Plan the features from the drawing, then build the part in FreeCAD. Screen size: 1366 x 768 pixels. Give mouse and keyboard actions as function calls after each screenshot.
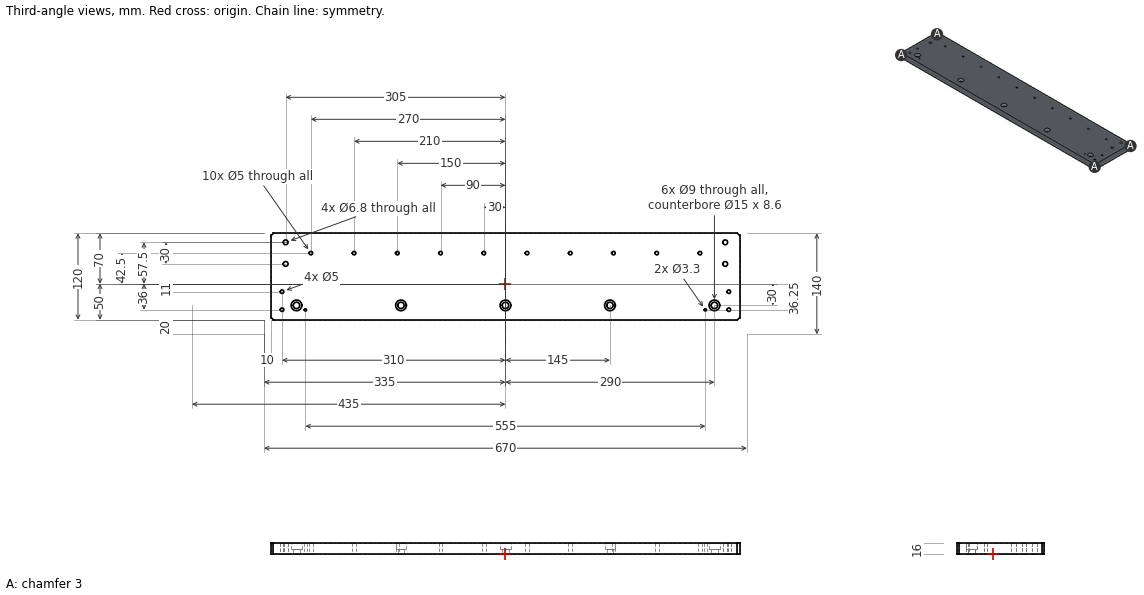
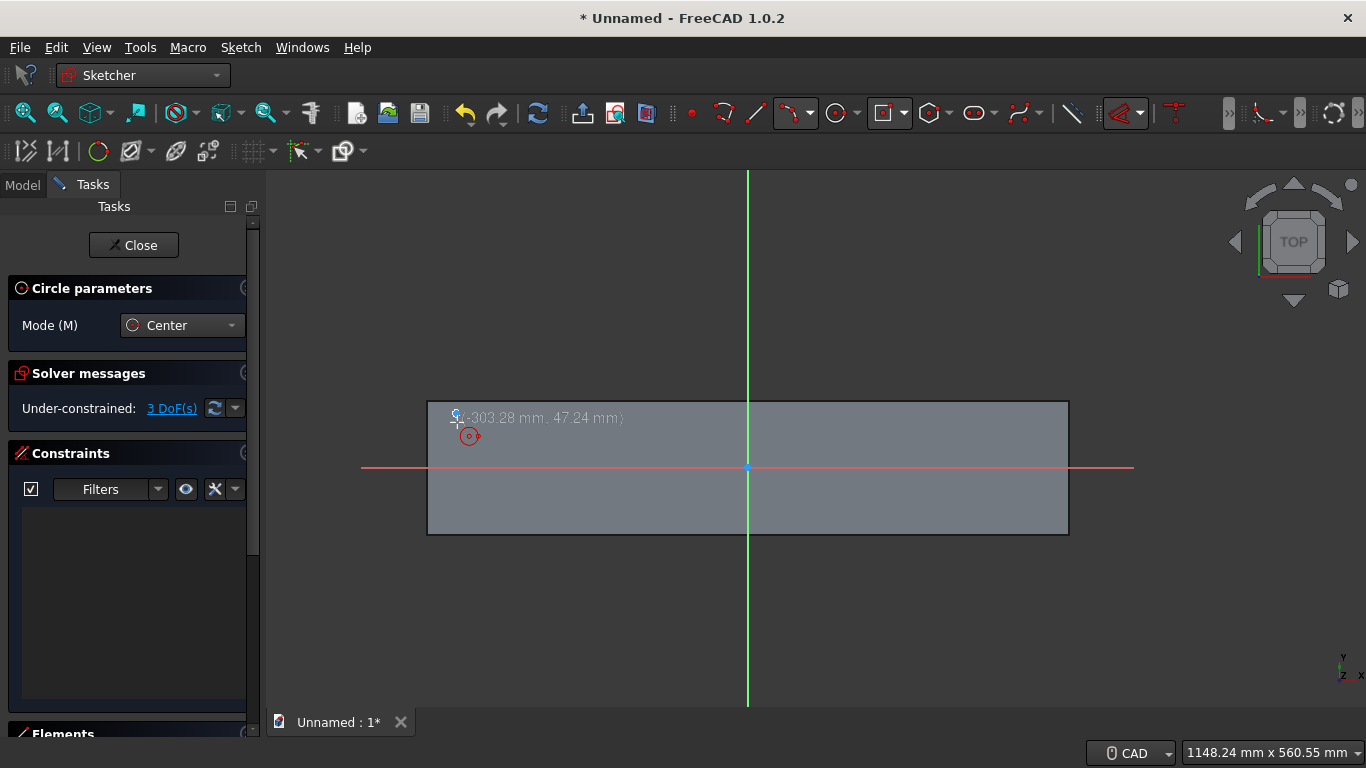
click(456, 441)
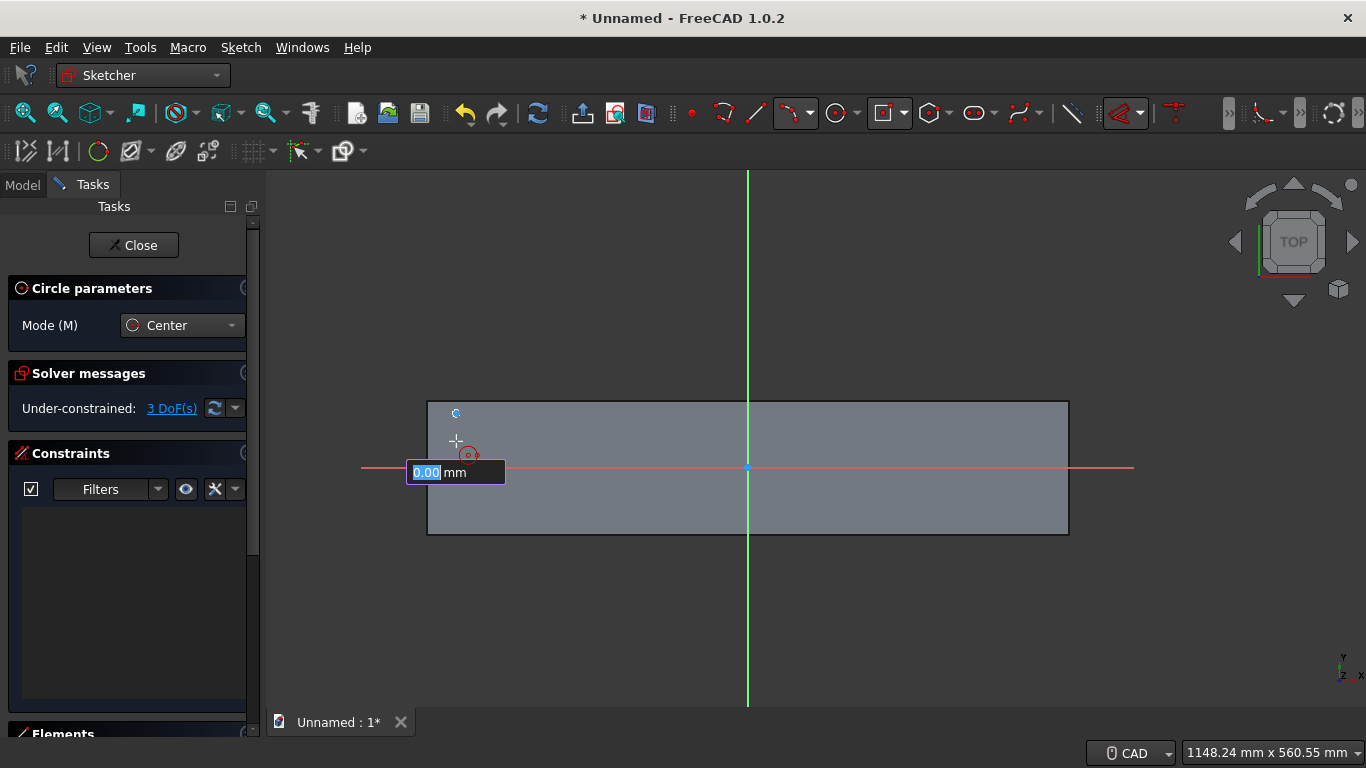
scroll(458, 439, up, 8)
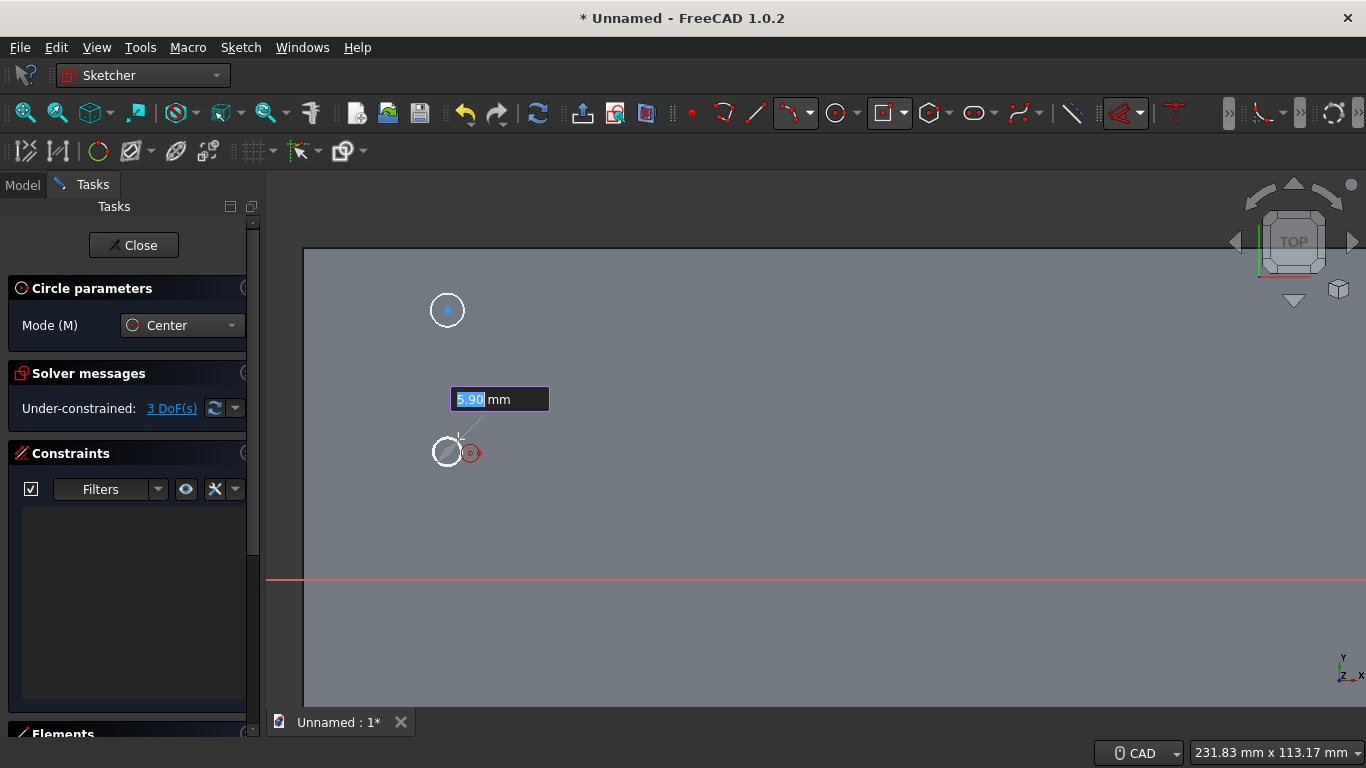
click(456, 438)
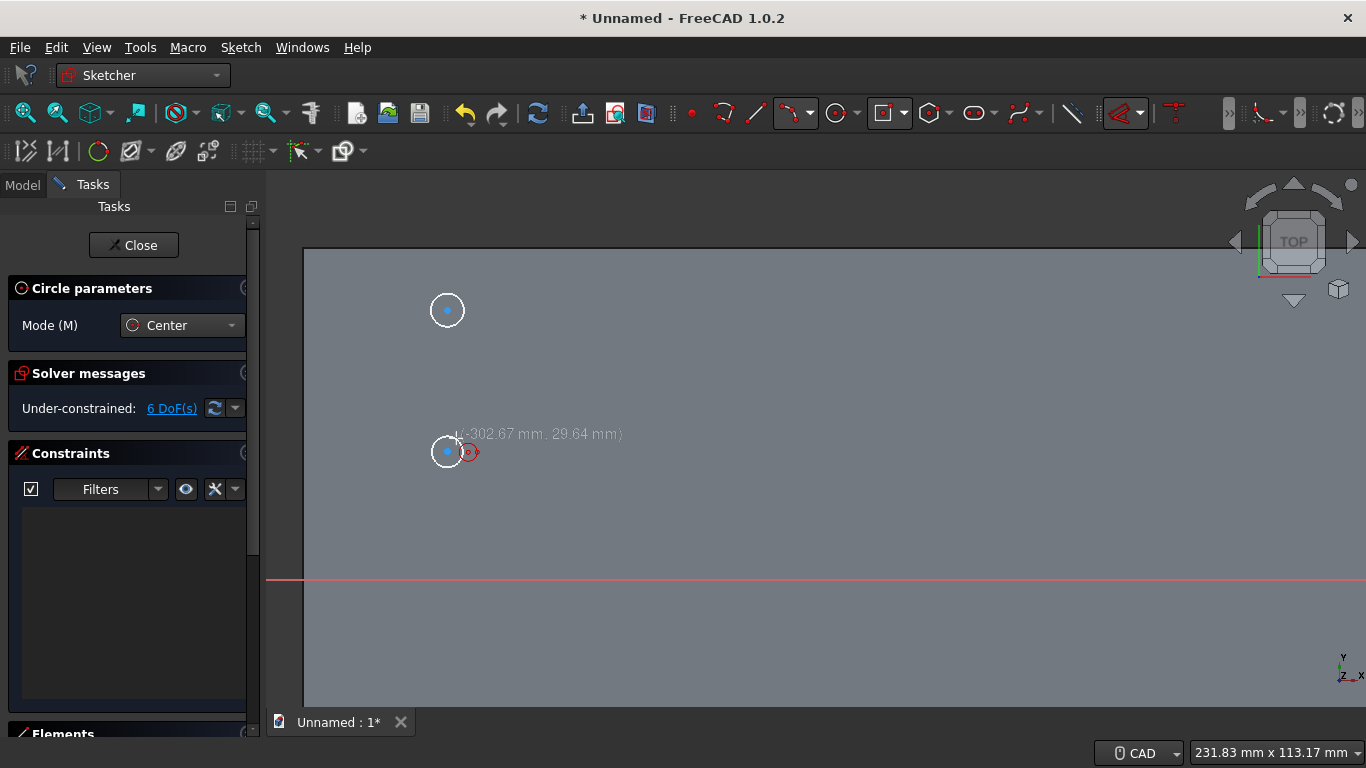
scroll(458, 439, down, 8)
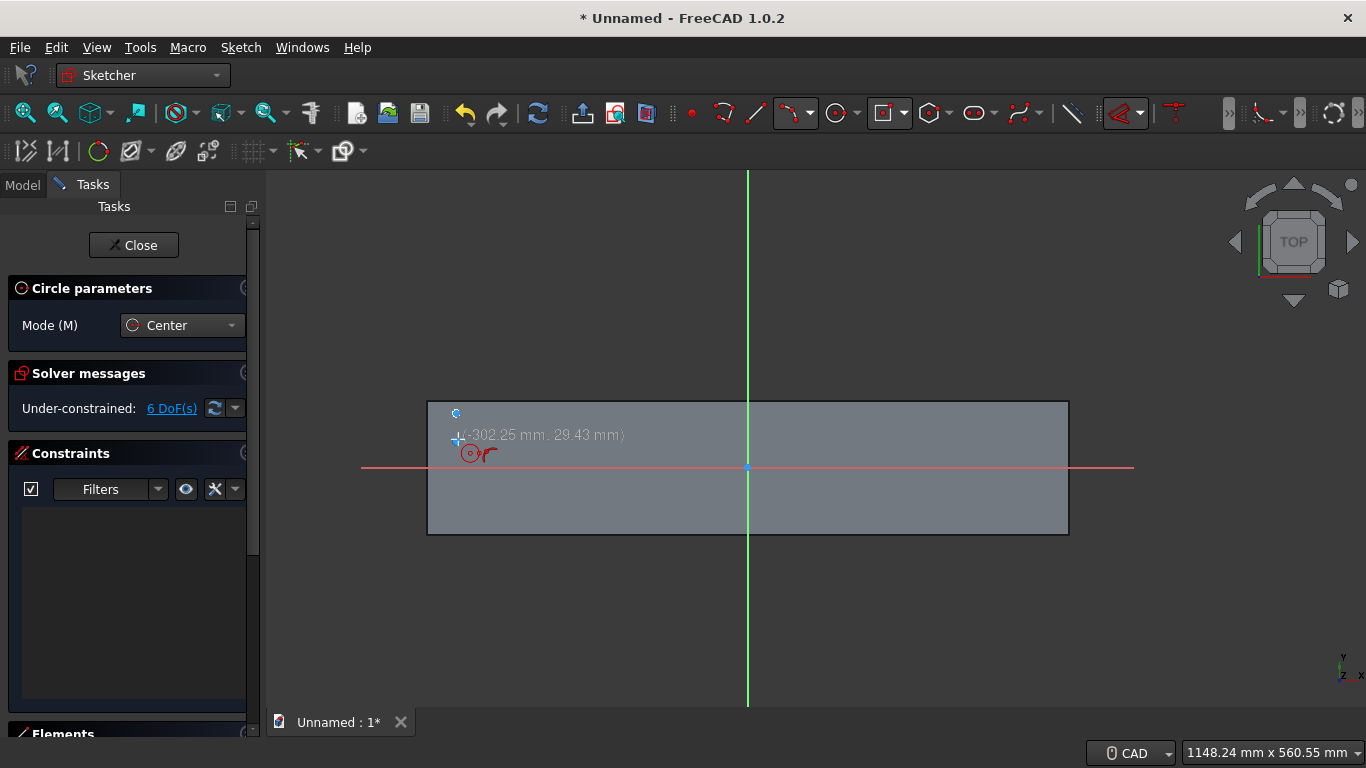
scroll(1040, 441, up, 10)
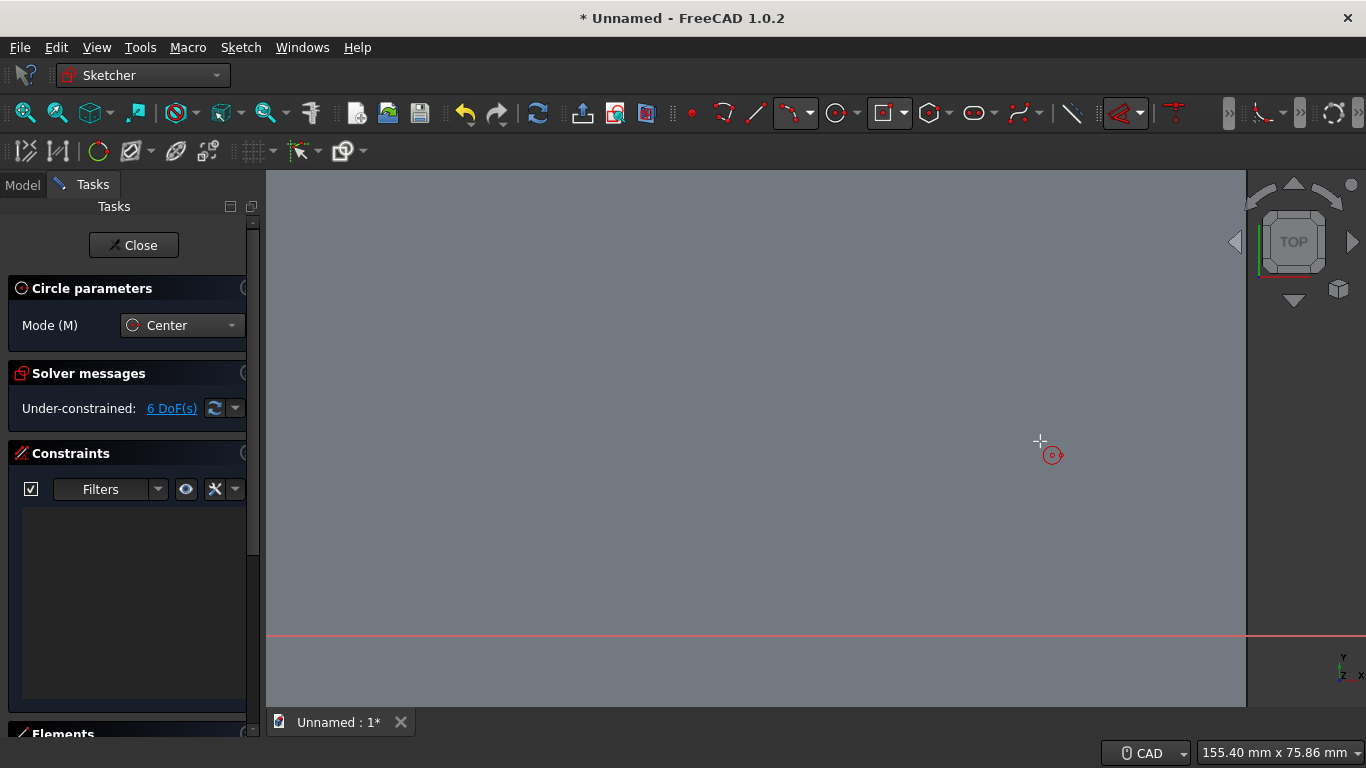
scroll(1040, 441, down, 10)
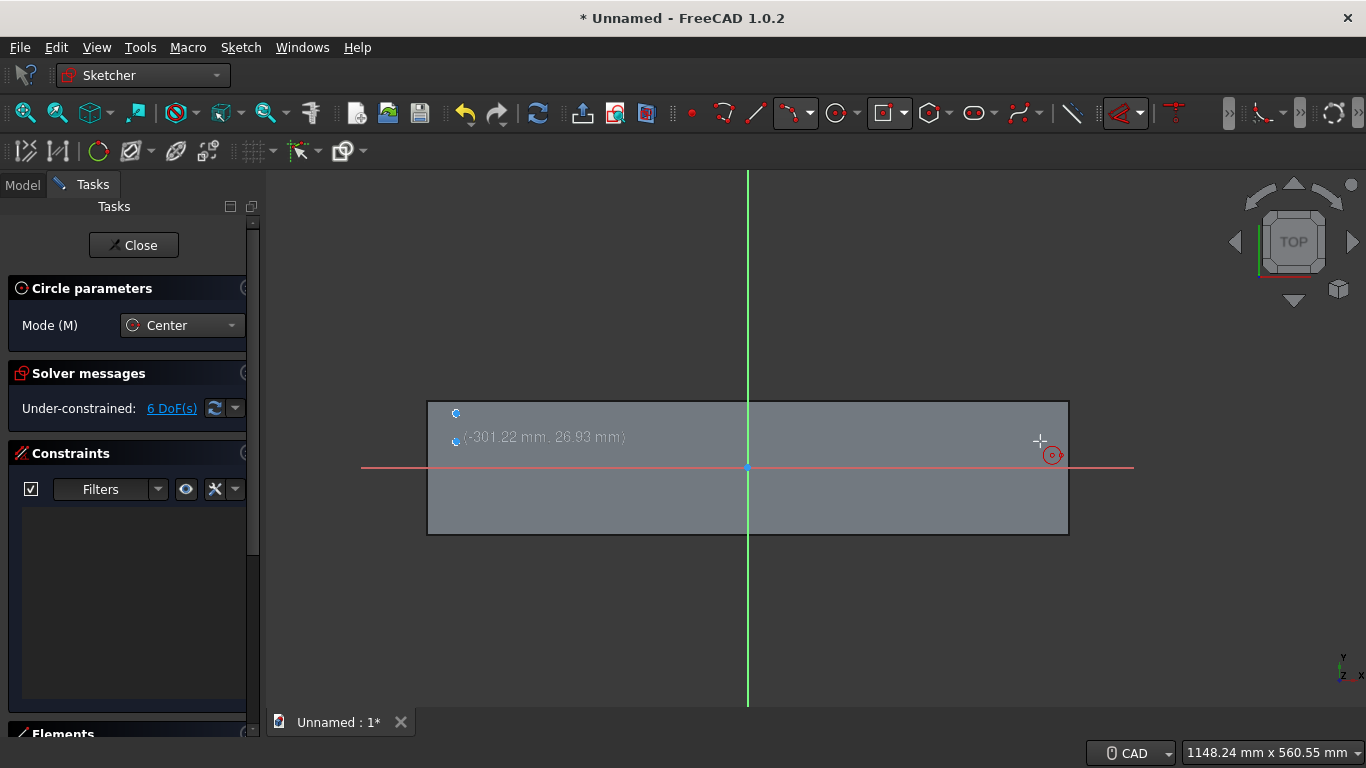
click(1040, 441)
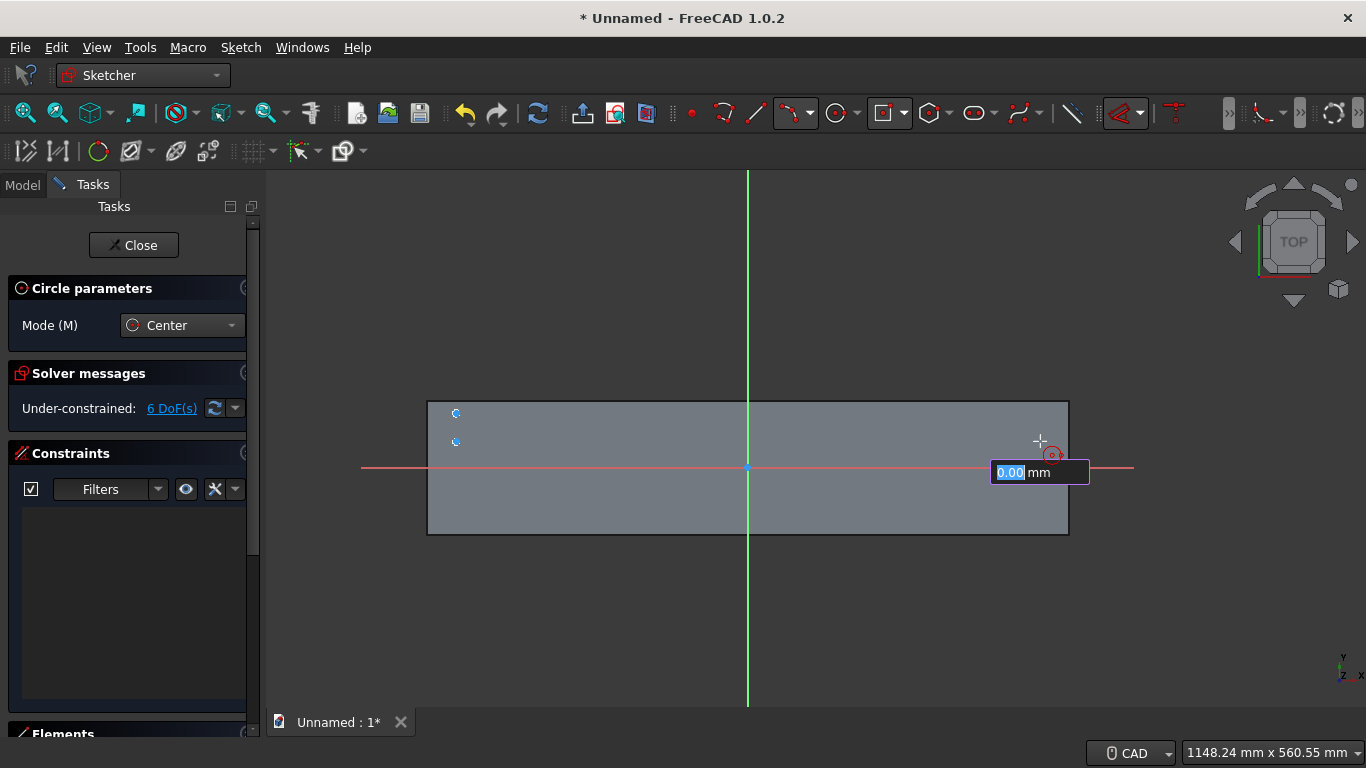
scroll(1042, 439, up, 8)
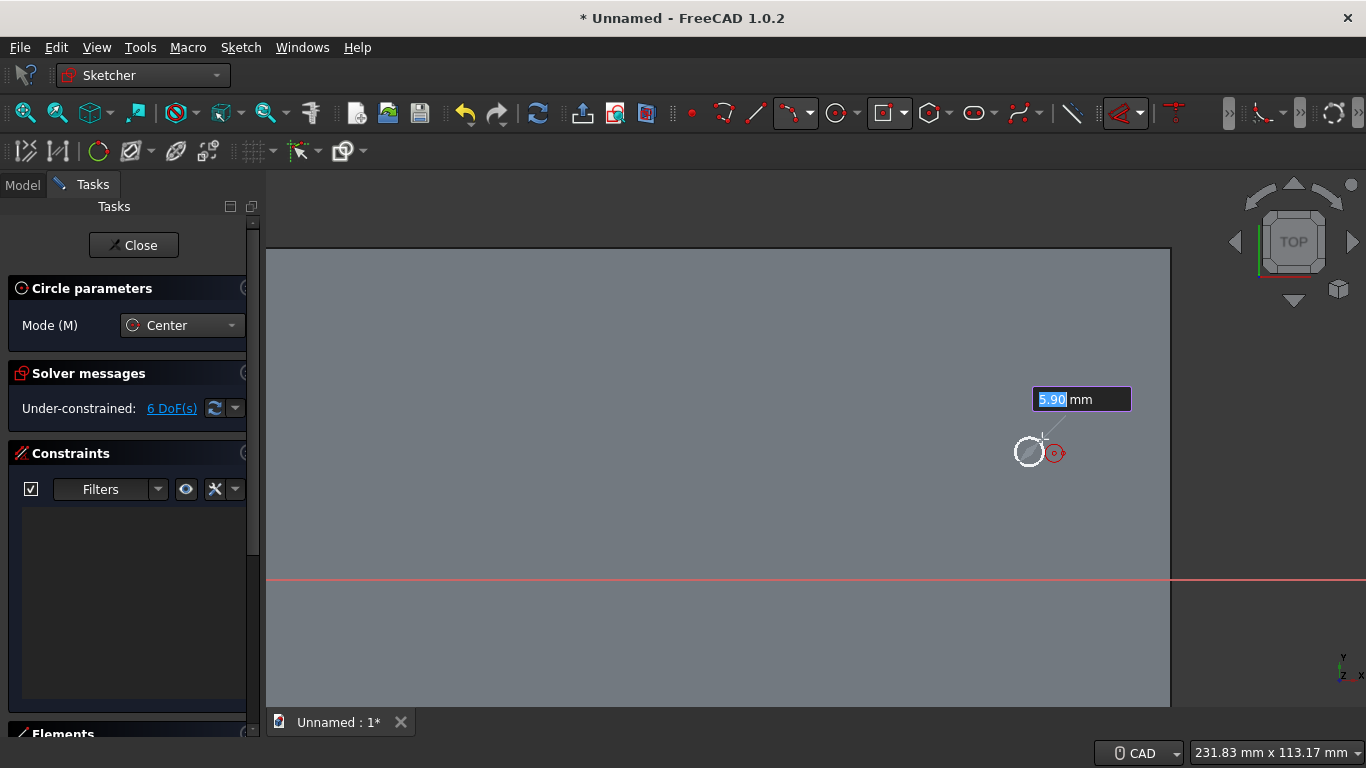
click(1040, 438)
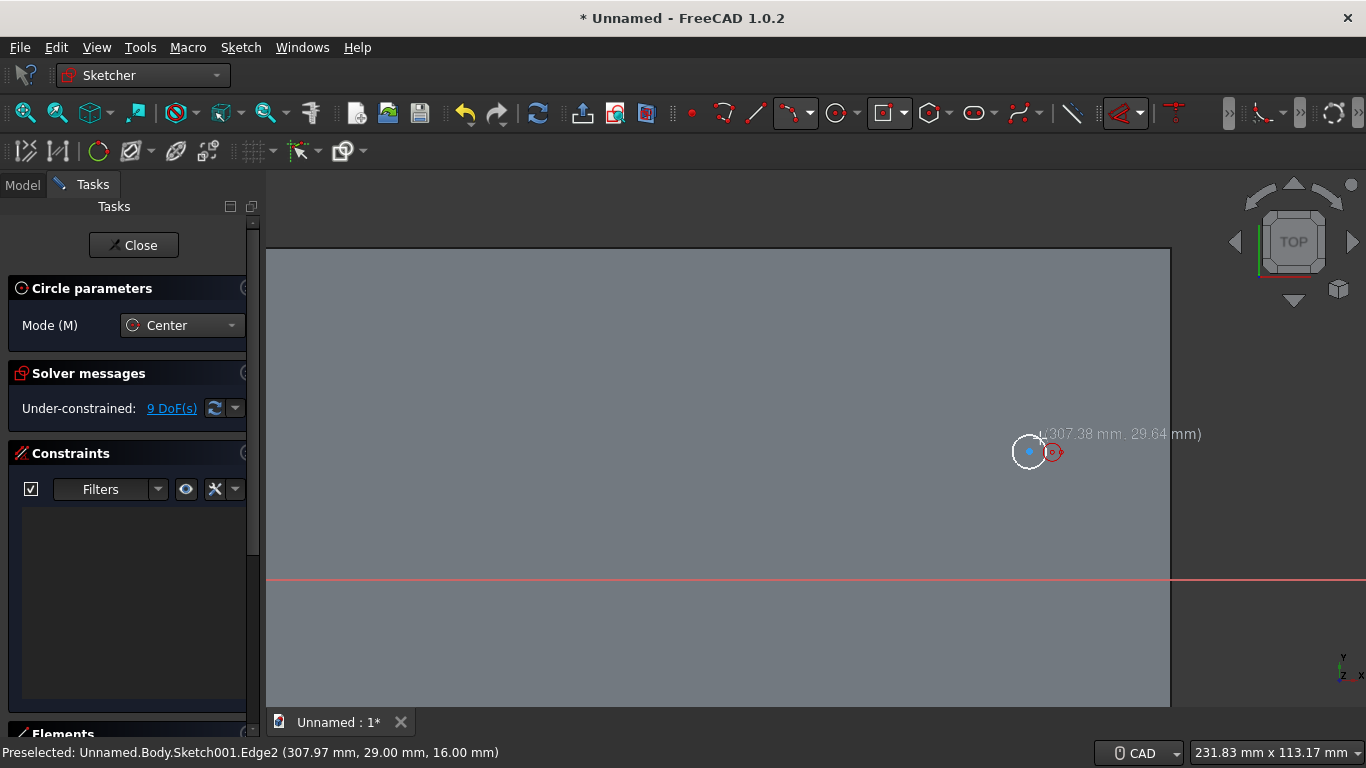
scroll(1029, 307, up, 2)